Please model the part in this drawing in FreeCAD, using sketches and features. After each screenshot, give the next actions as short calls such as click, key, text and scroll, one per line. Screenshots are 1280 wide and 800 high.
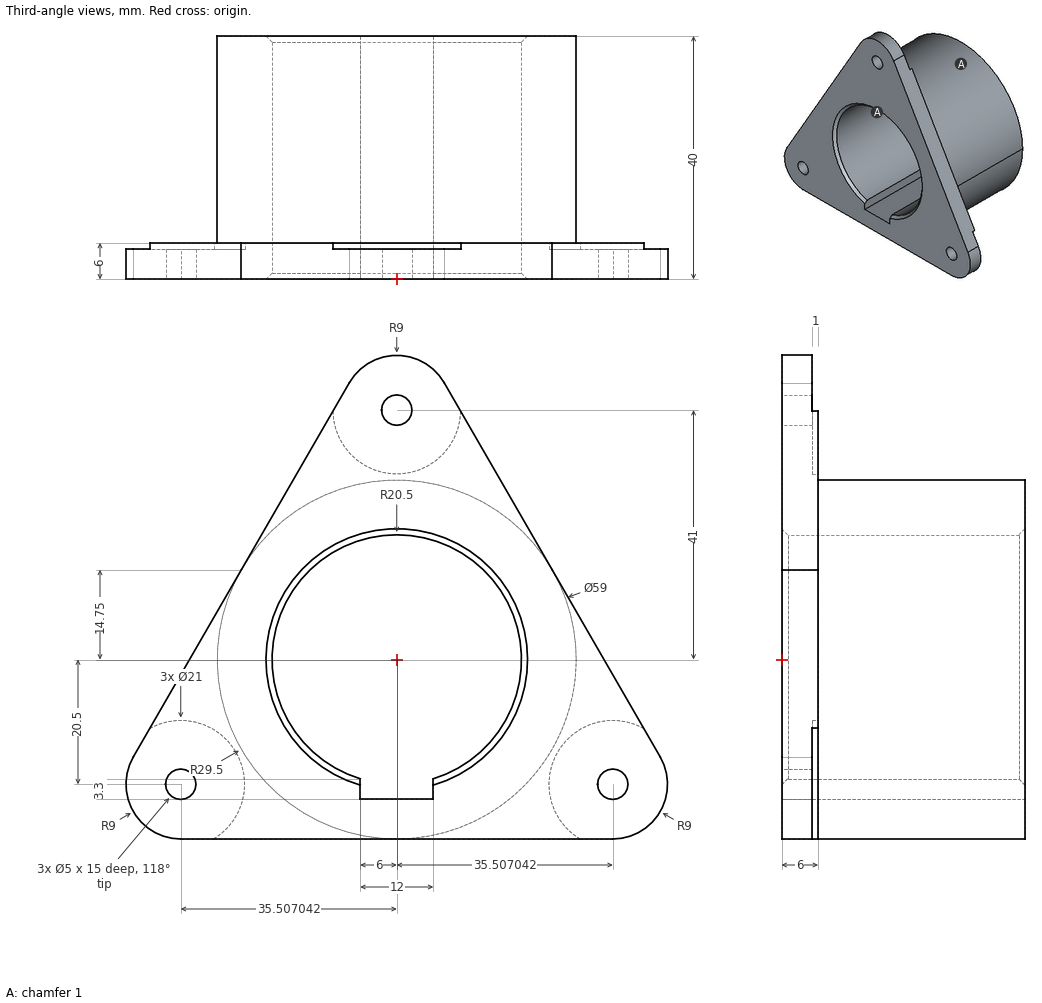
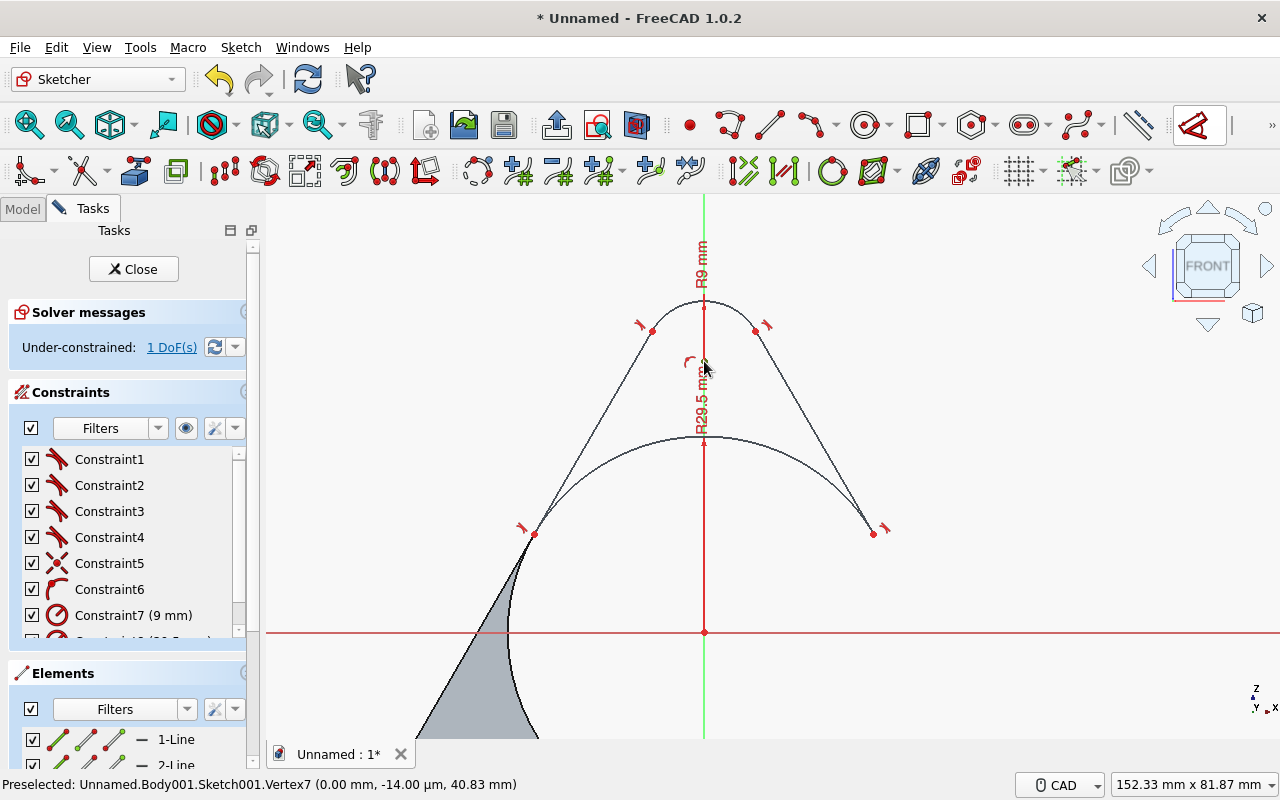
click(1220, 126)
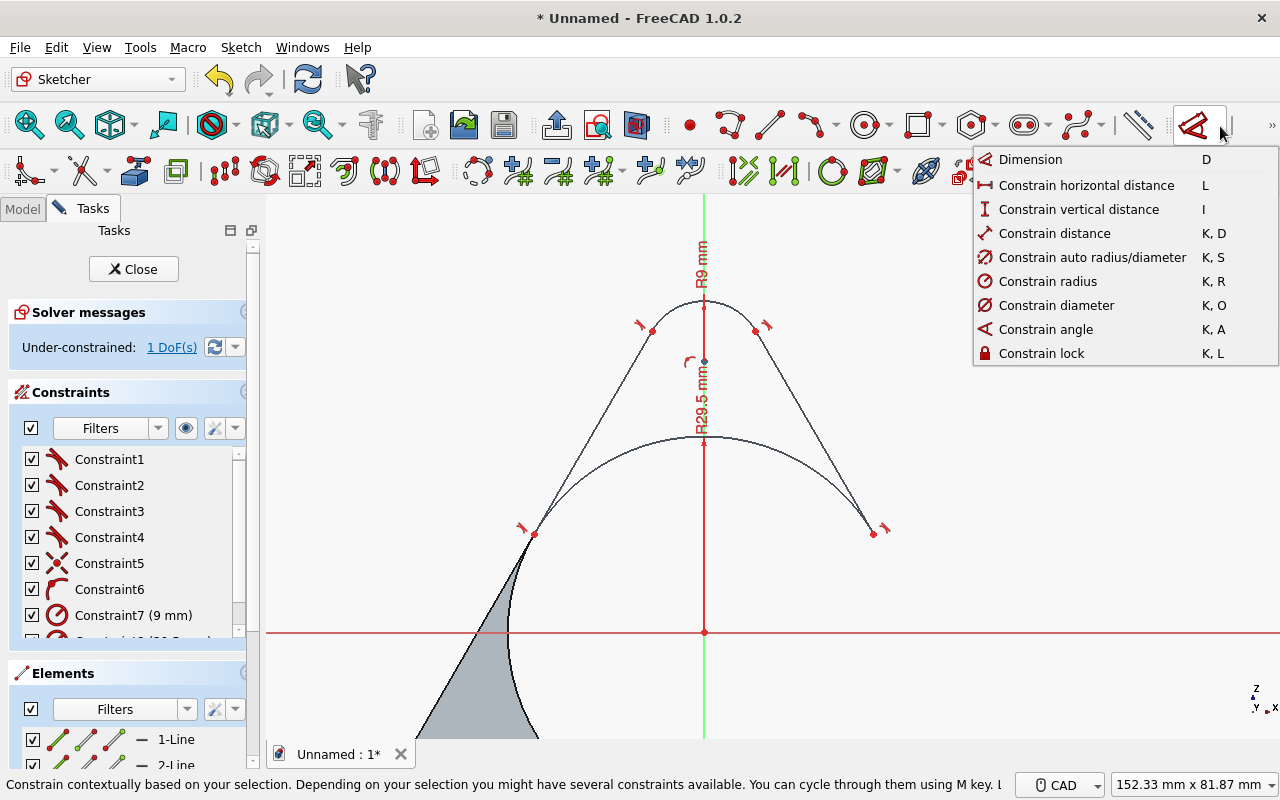
click(1126, 209)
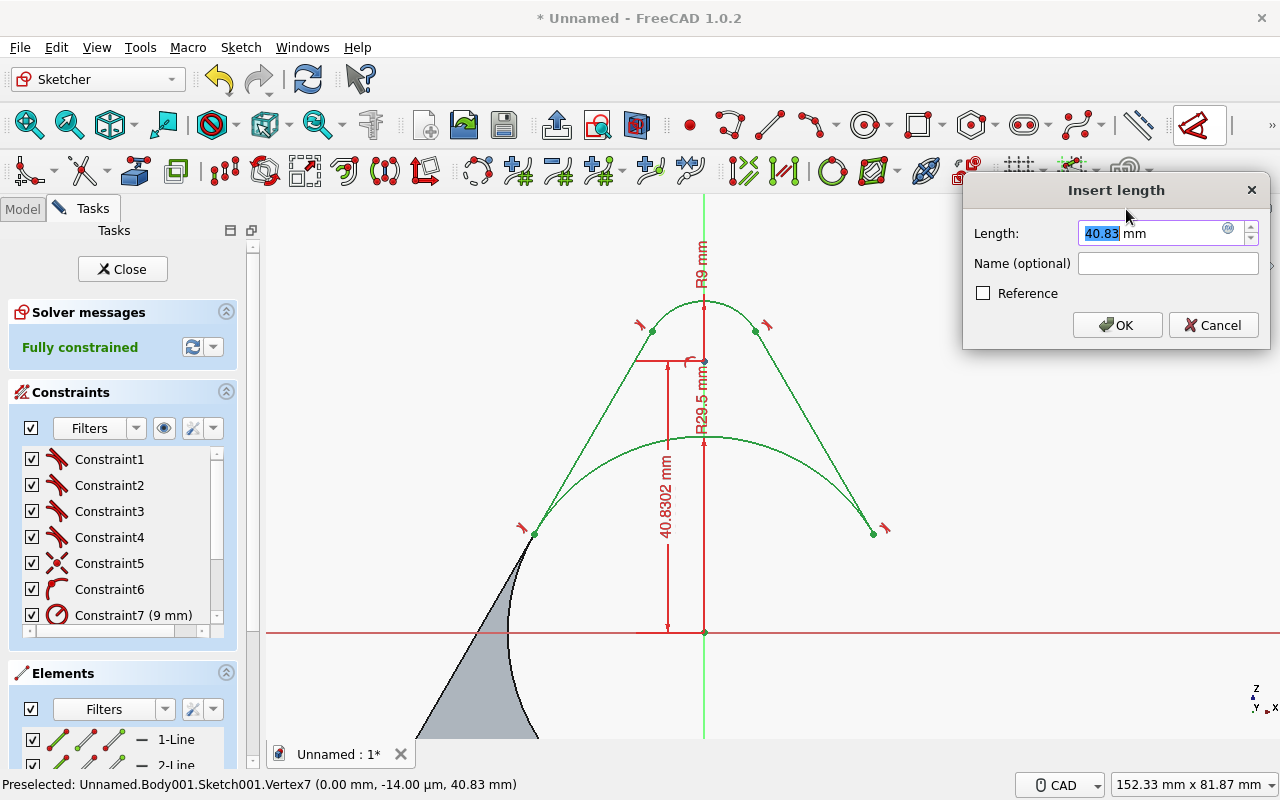
text(41)
key(Return)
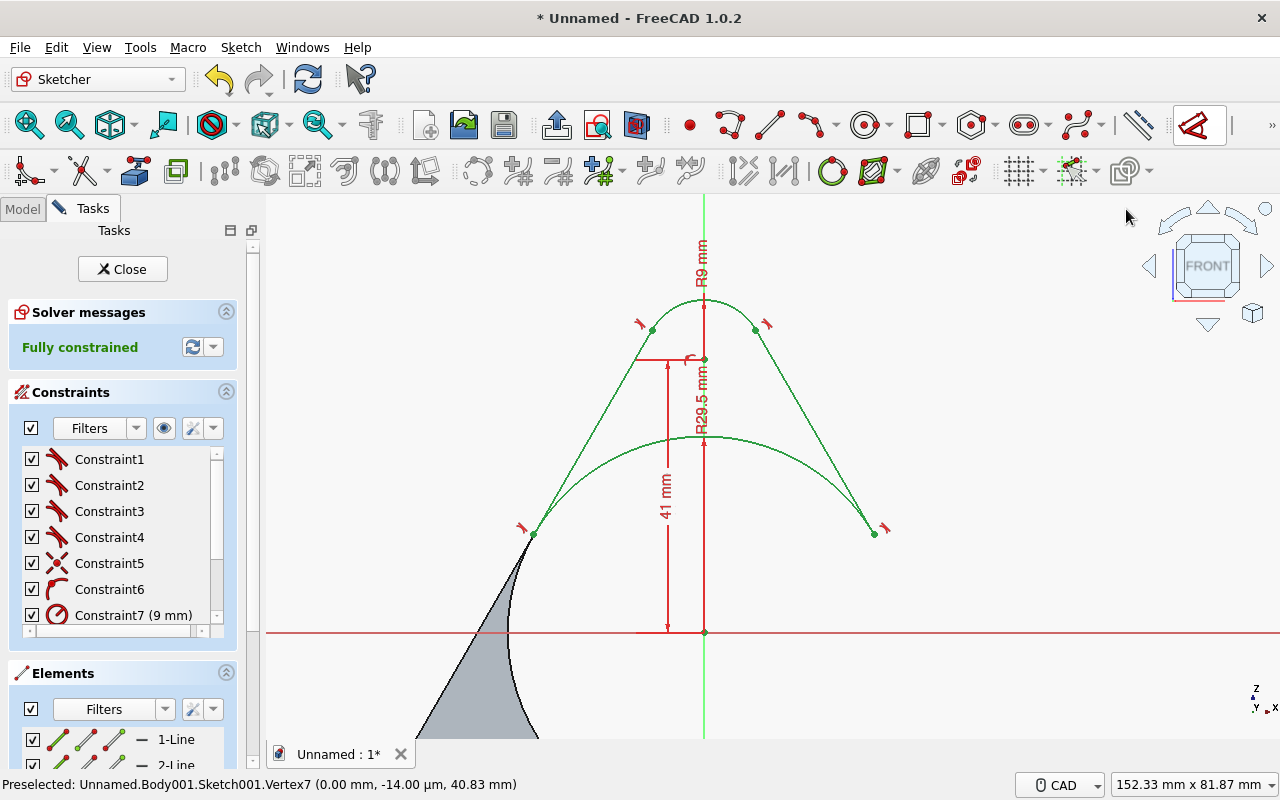
click(123, 269)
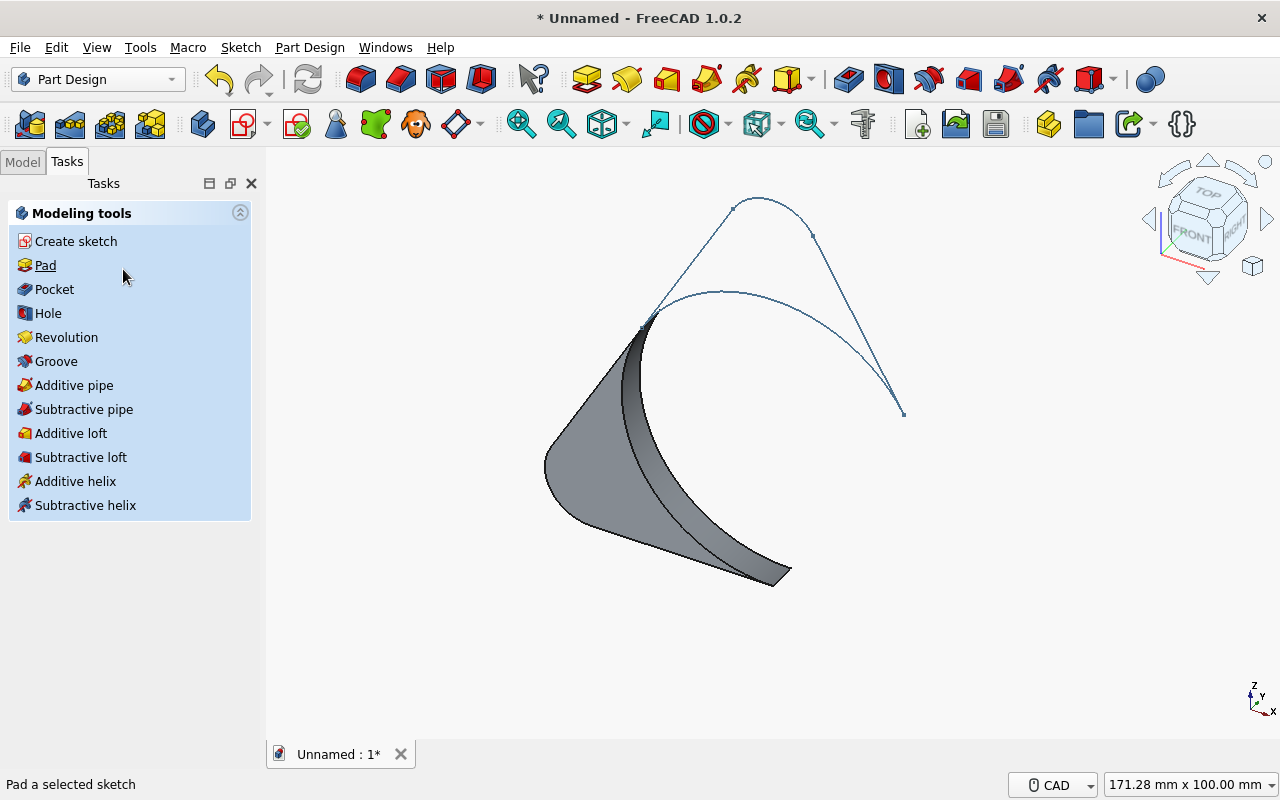
click(588, 80)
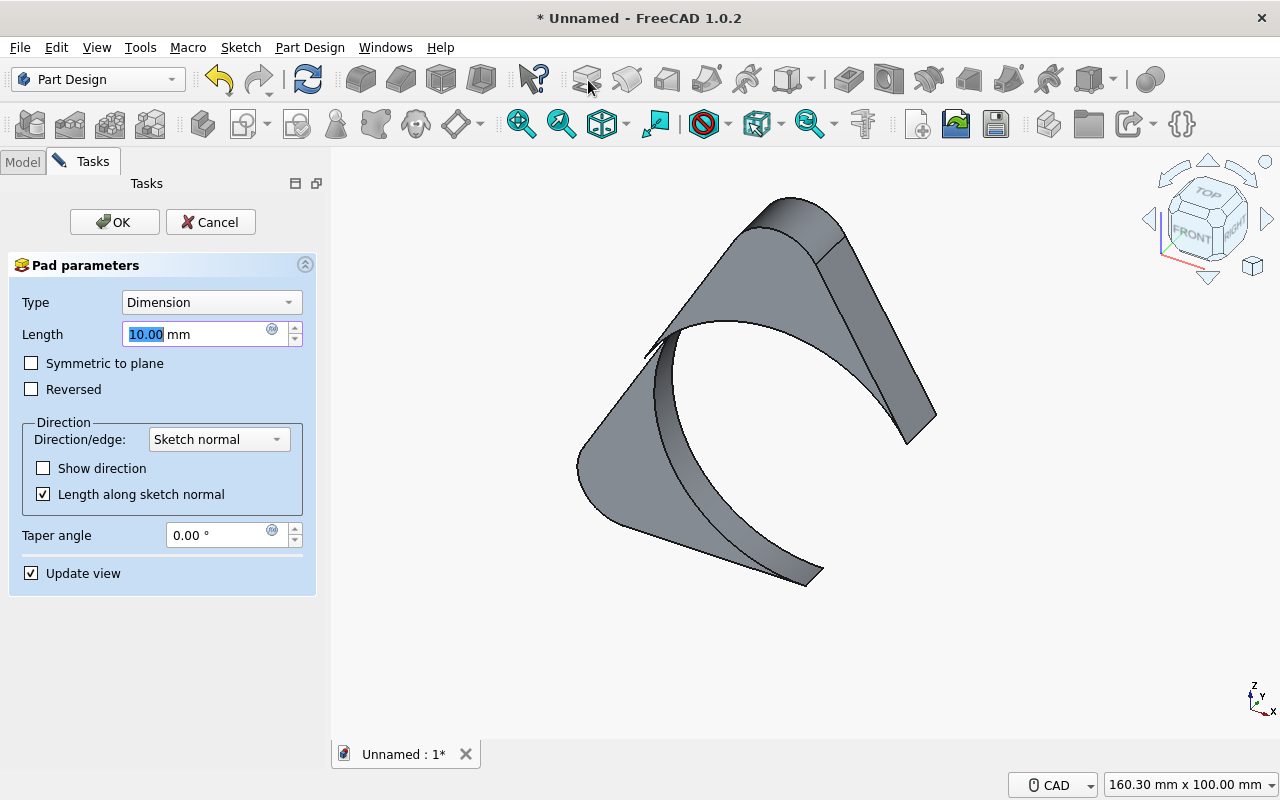
text(6)
key(Tab)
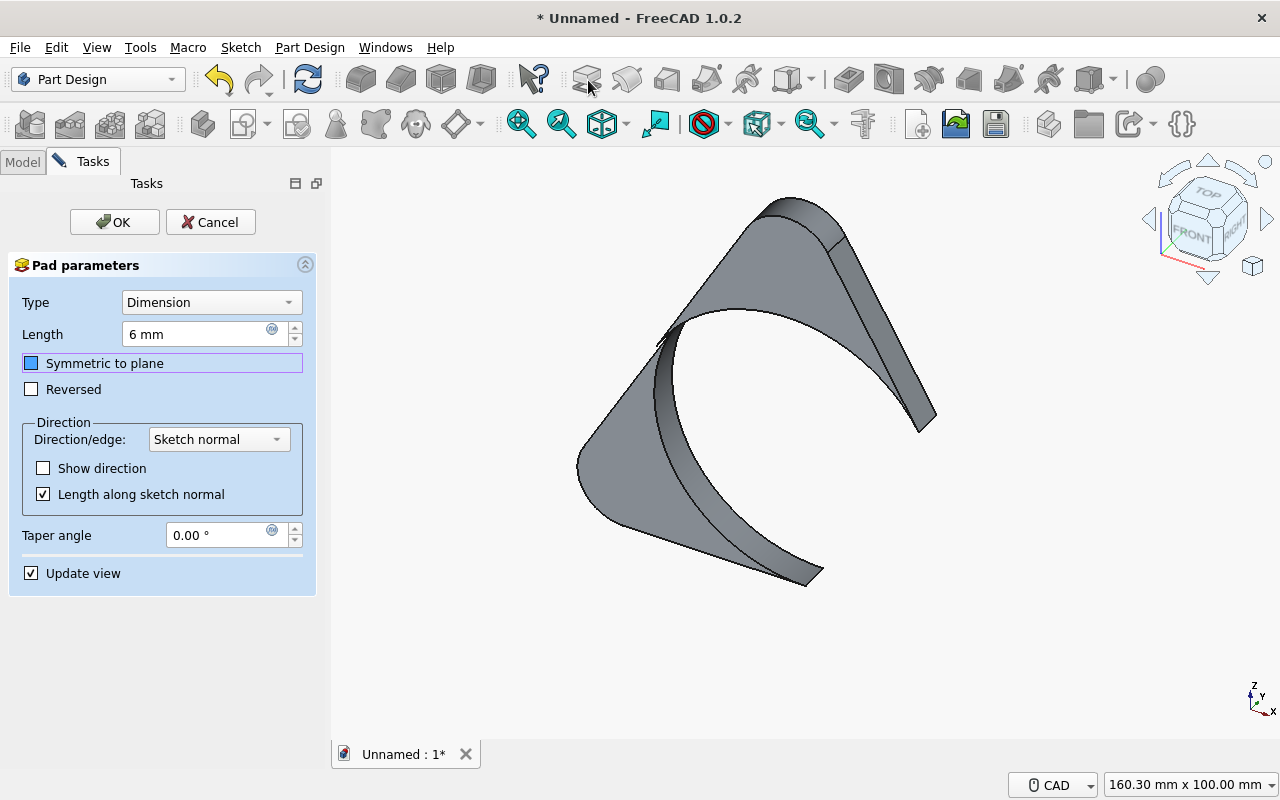
click(30, 389)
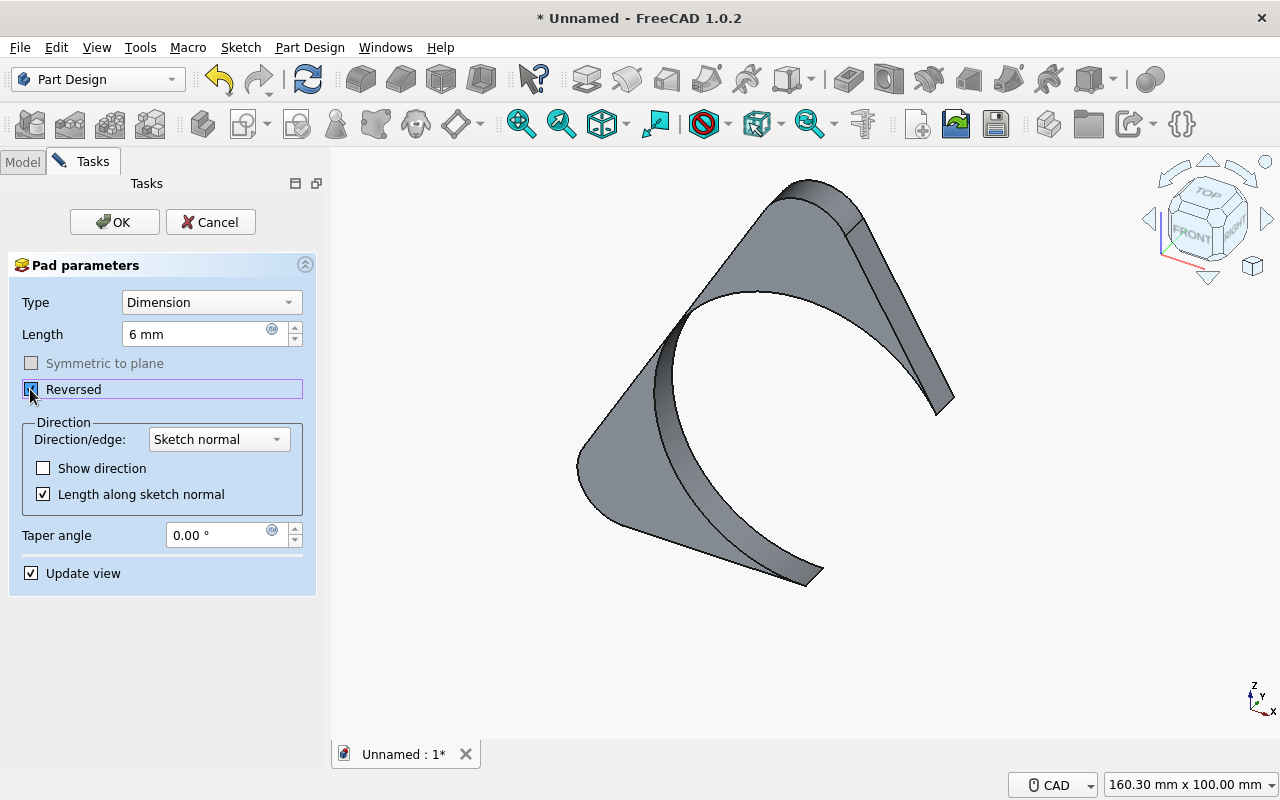
click(115, 222)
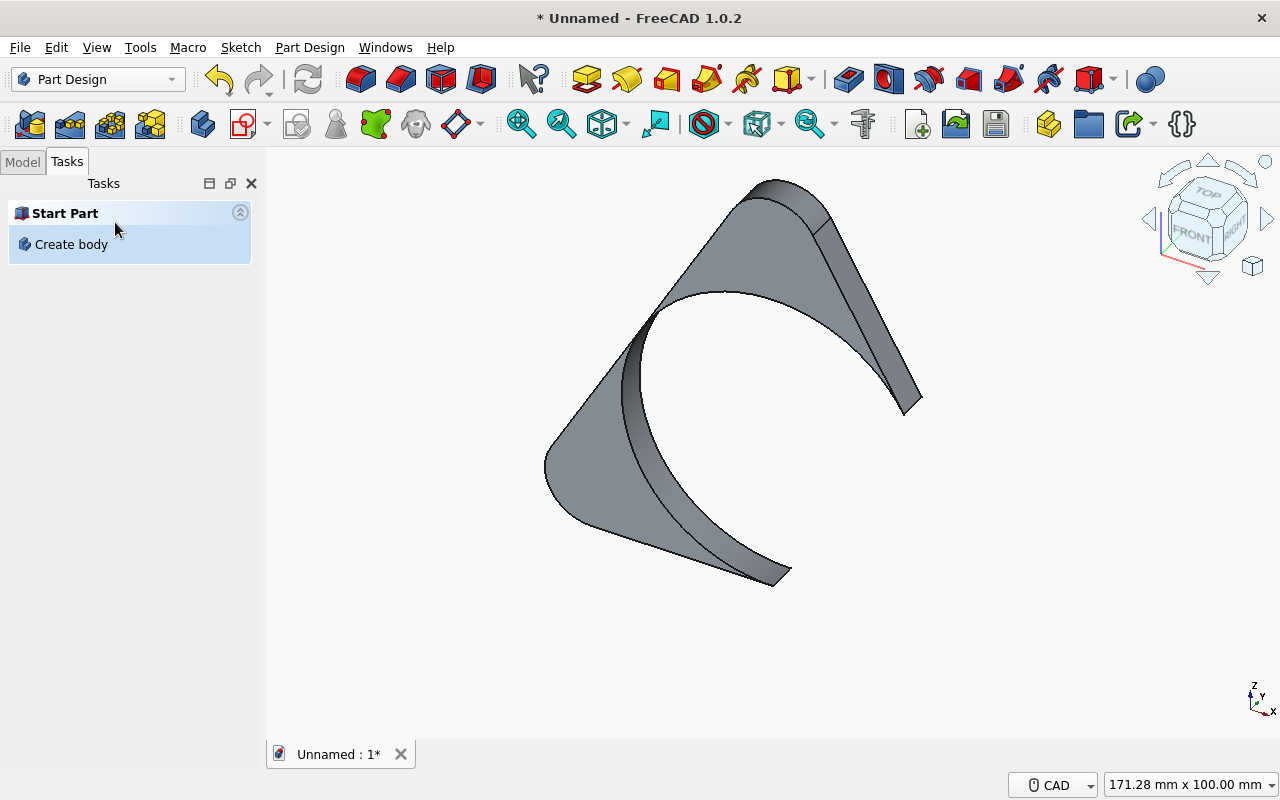
click(522, 124)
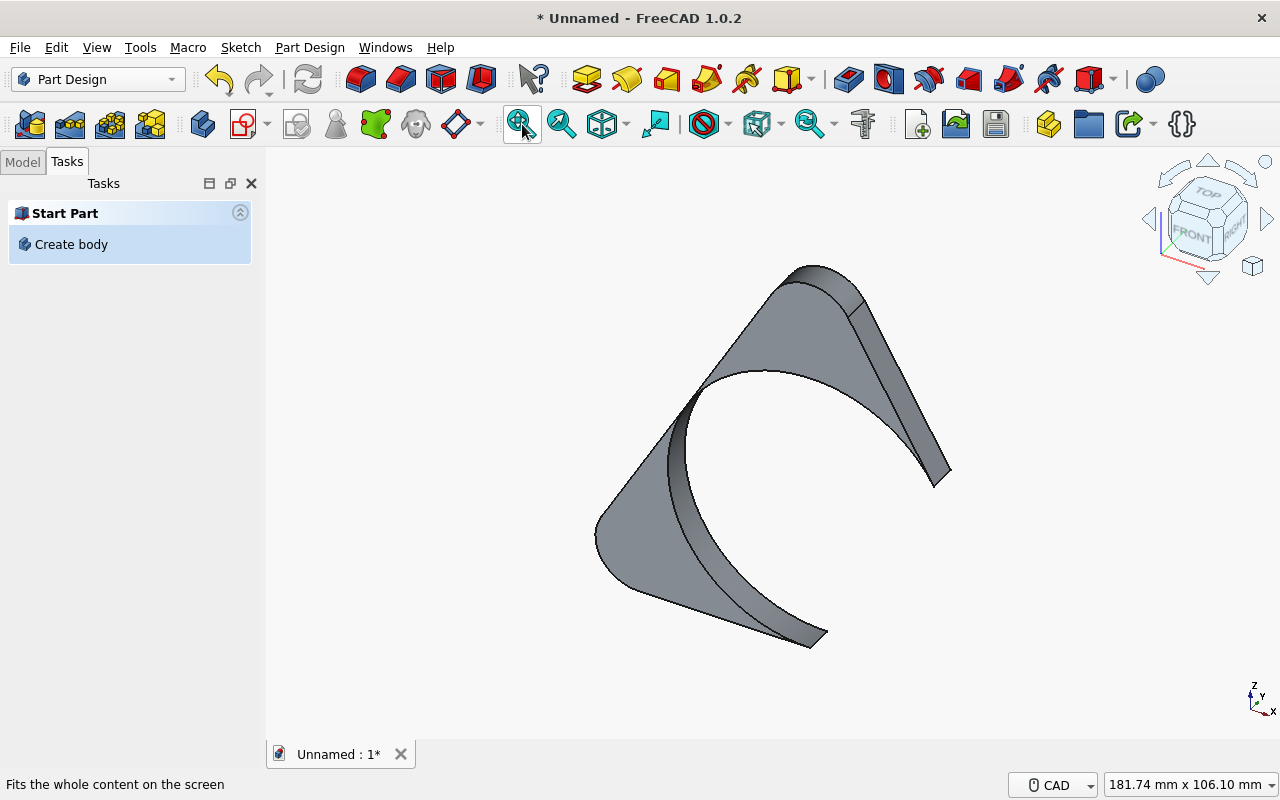
click(204, 124)